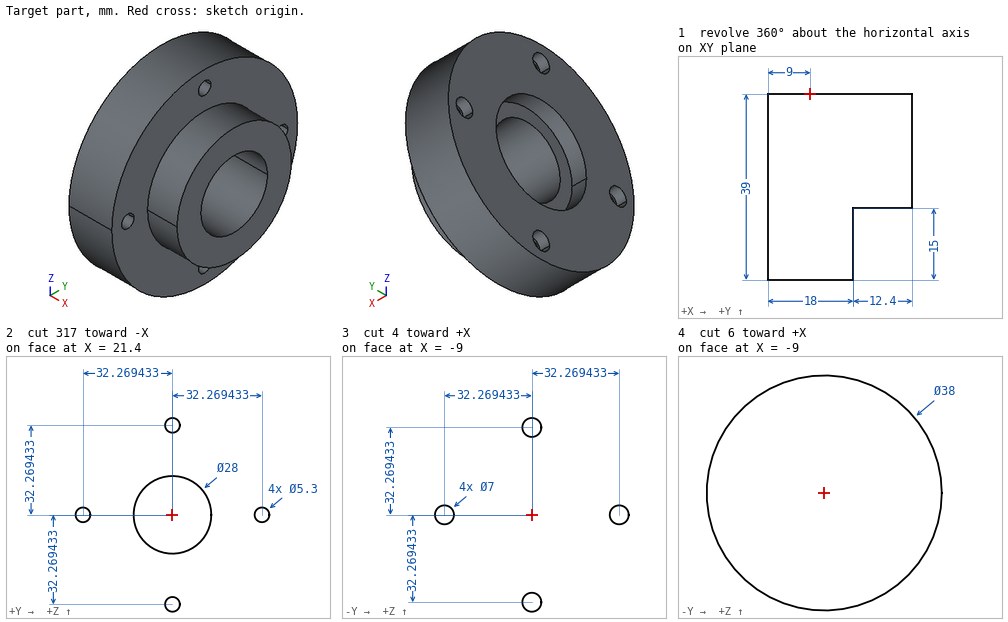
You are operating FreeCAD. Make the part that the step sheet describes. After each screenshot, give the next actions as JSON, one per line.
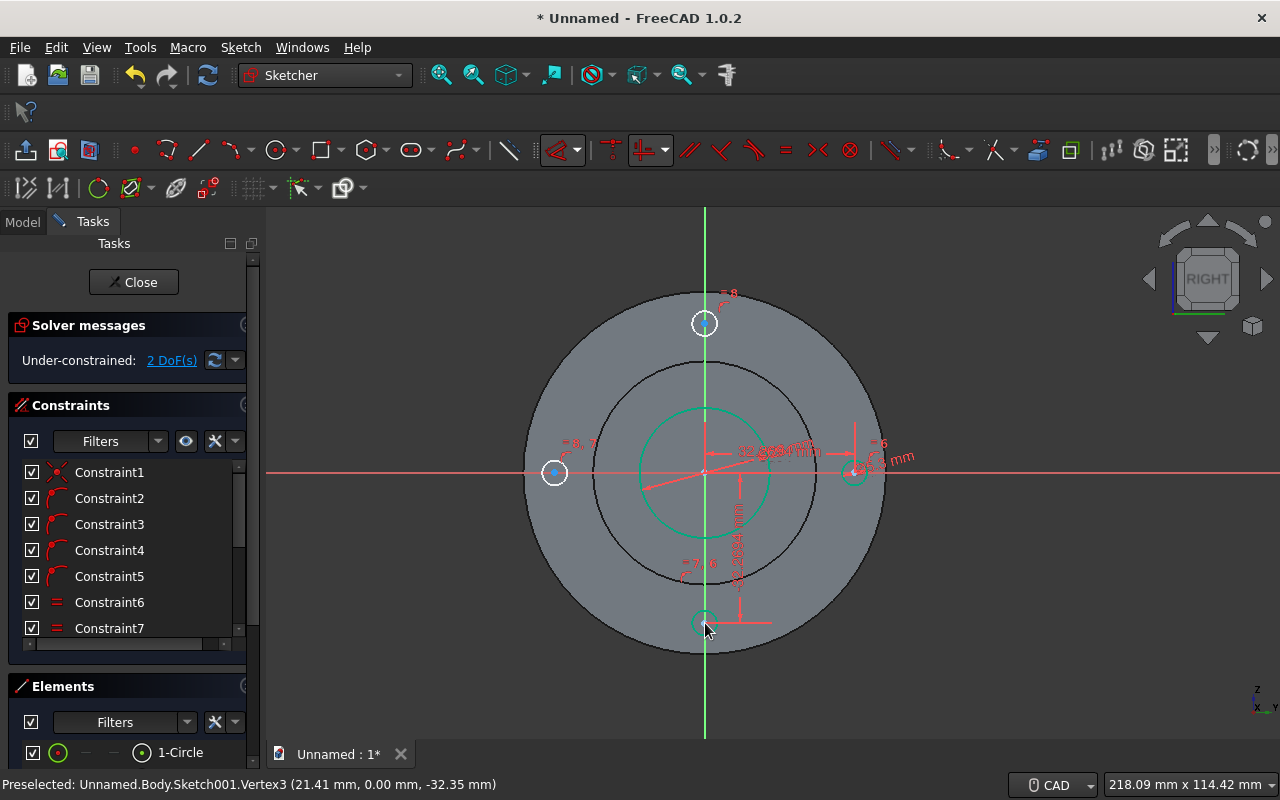
{"action": "left_click", "coordinate": [555, 473]}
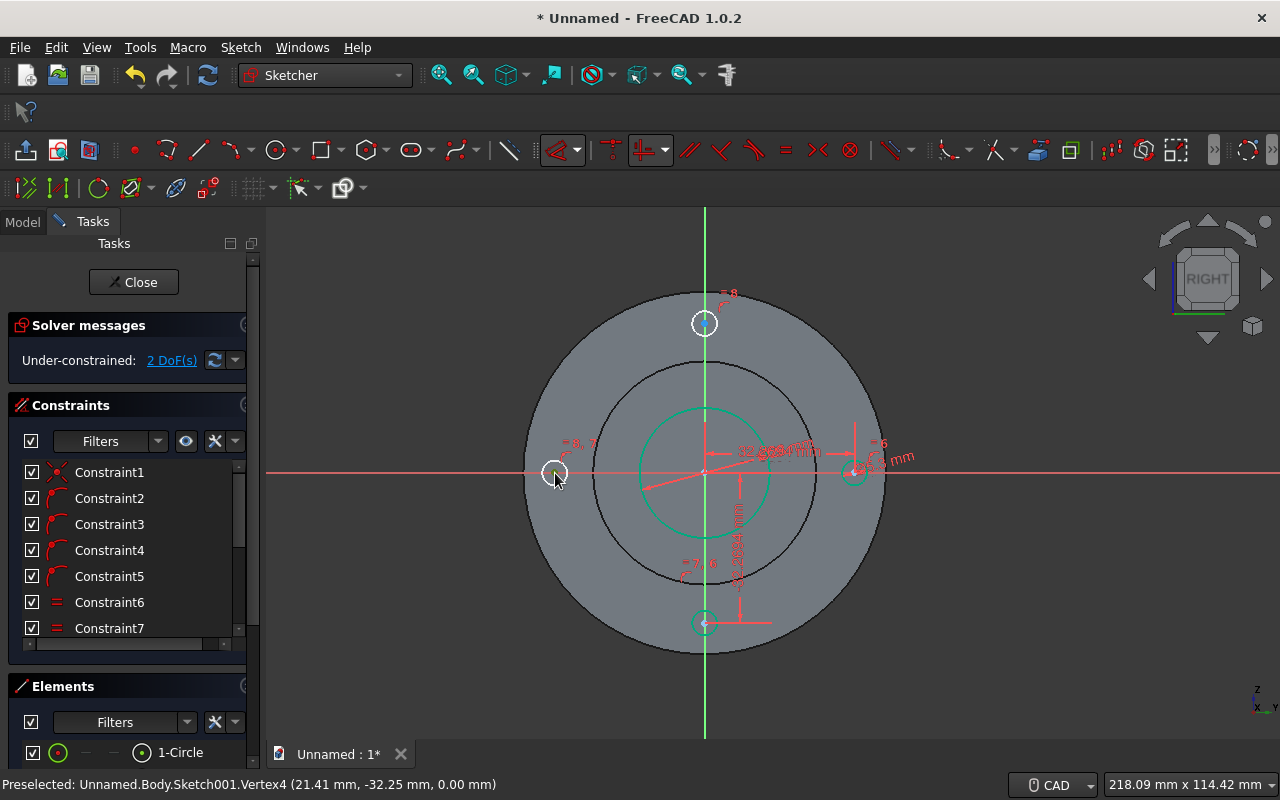
{"action": "left_click", "coordinate": [580, 150]}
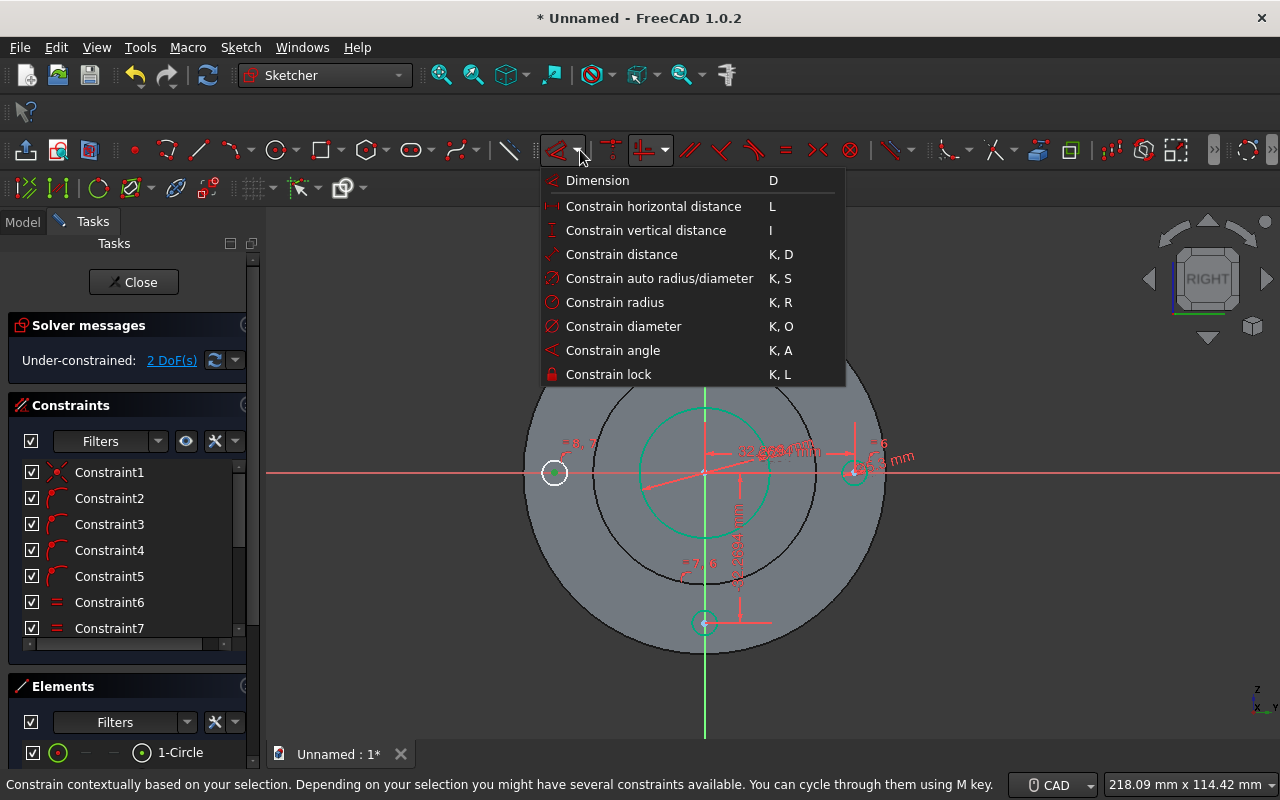
{"action": "left_click", "coordinate": [693, 206]}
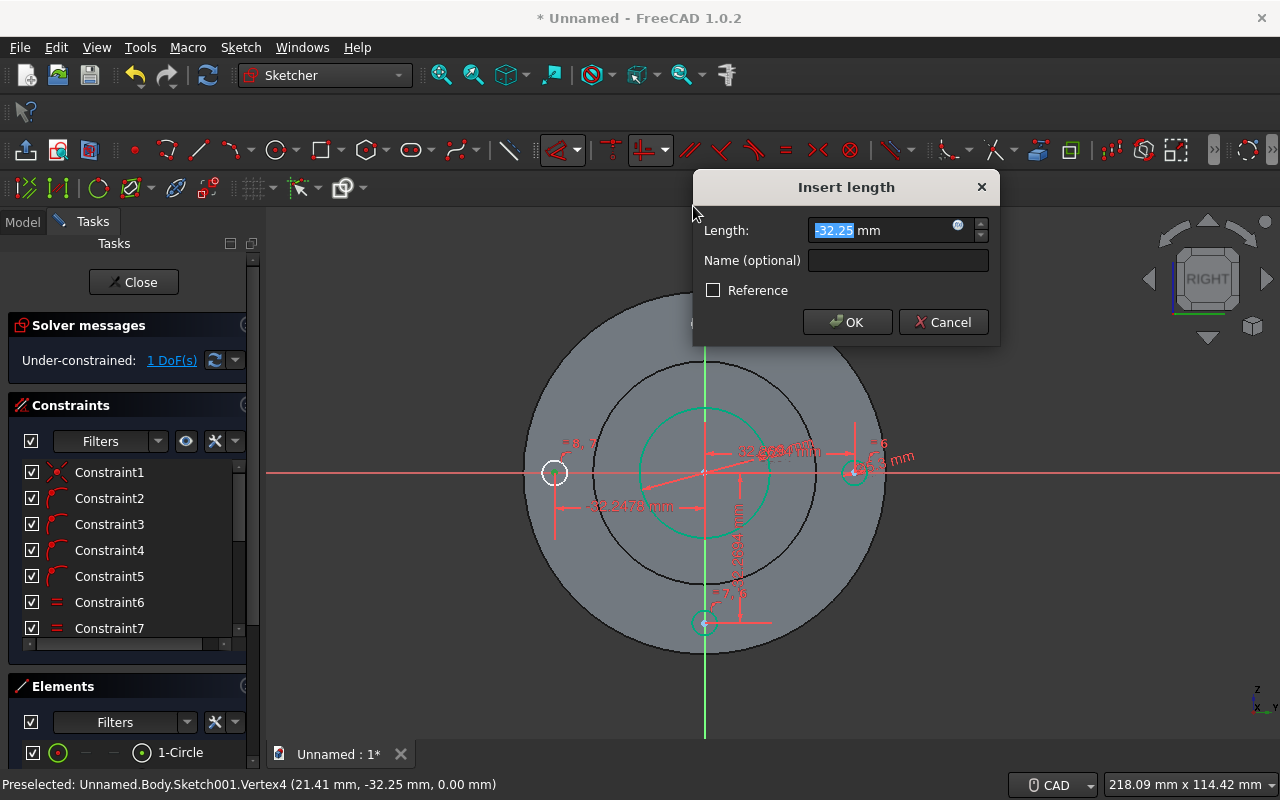
{"action": "type", "text": "-32.269433"}
{"action": "key", "text": "Return"}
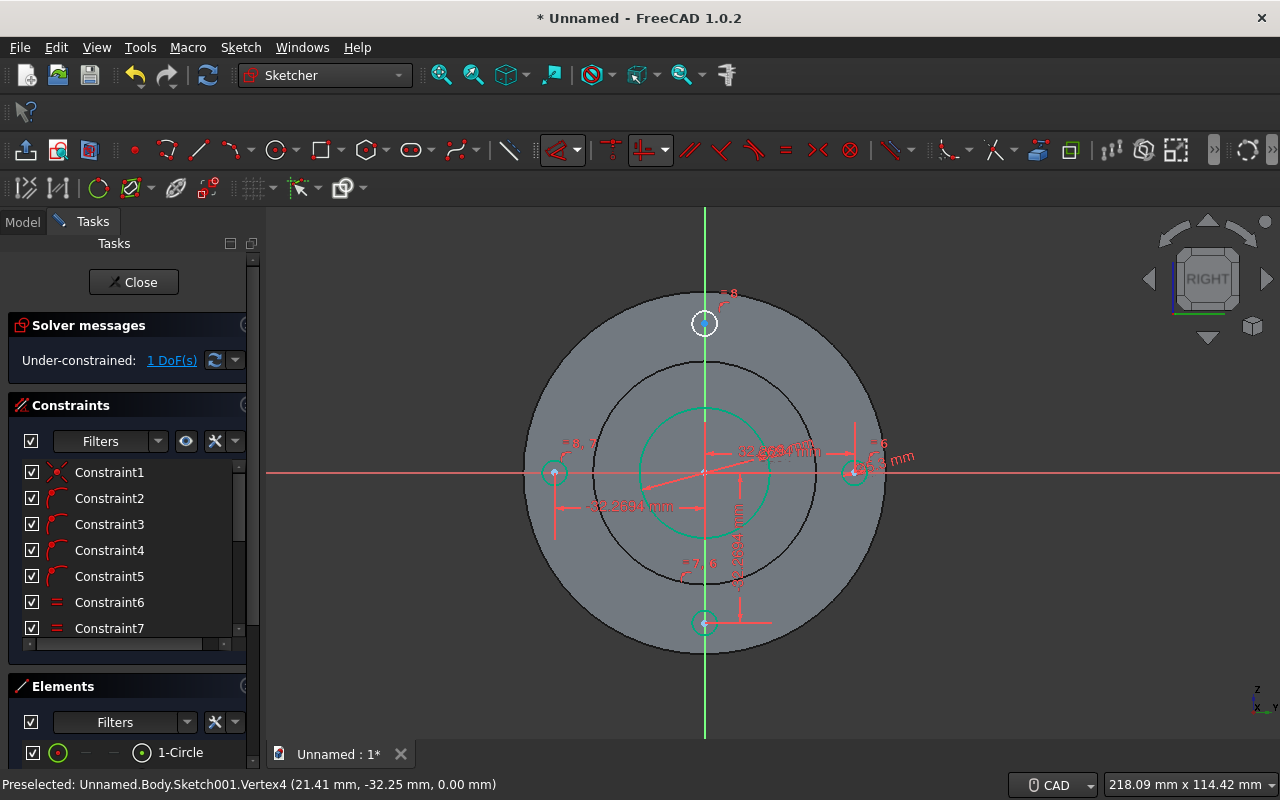
{"action": "left_click", "coordinate": [705, 324]}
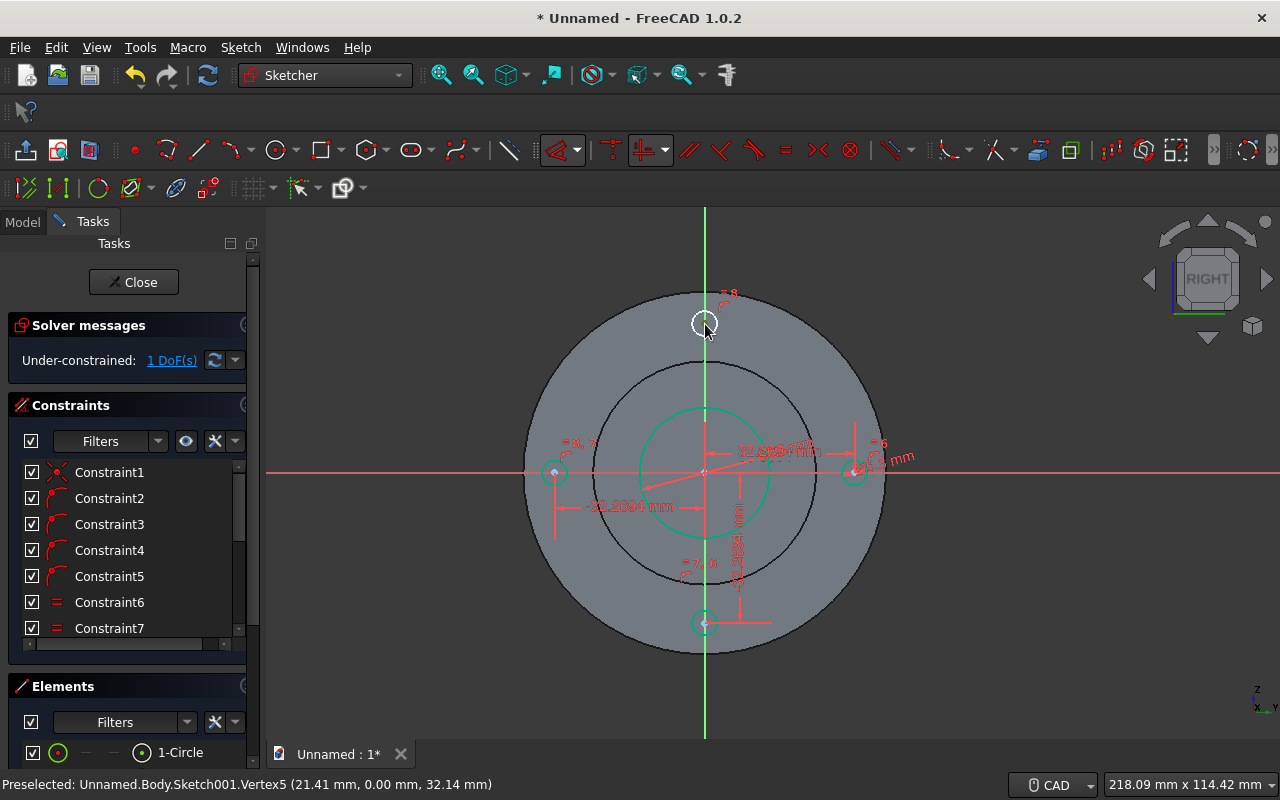
{"action": "left_click", "coordinate": [580, 150]}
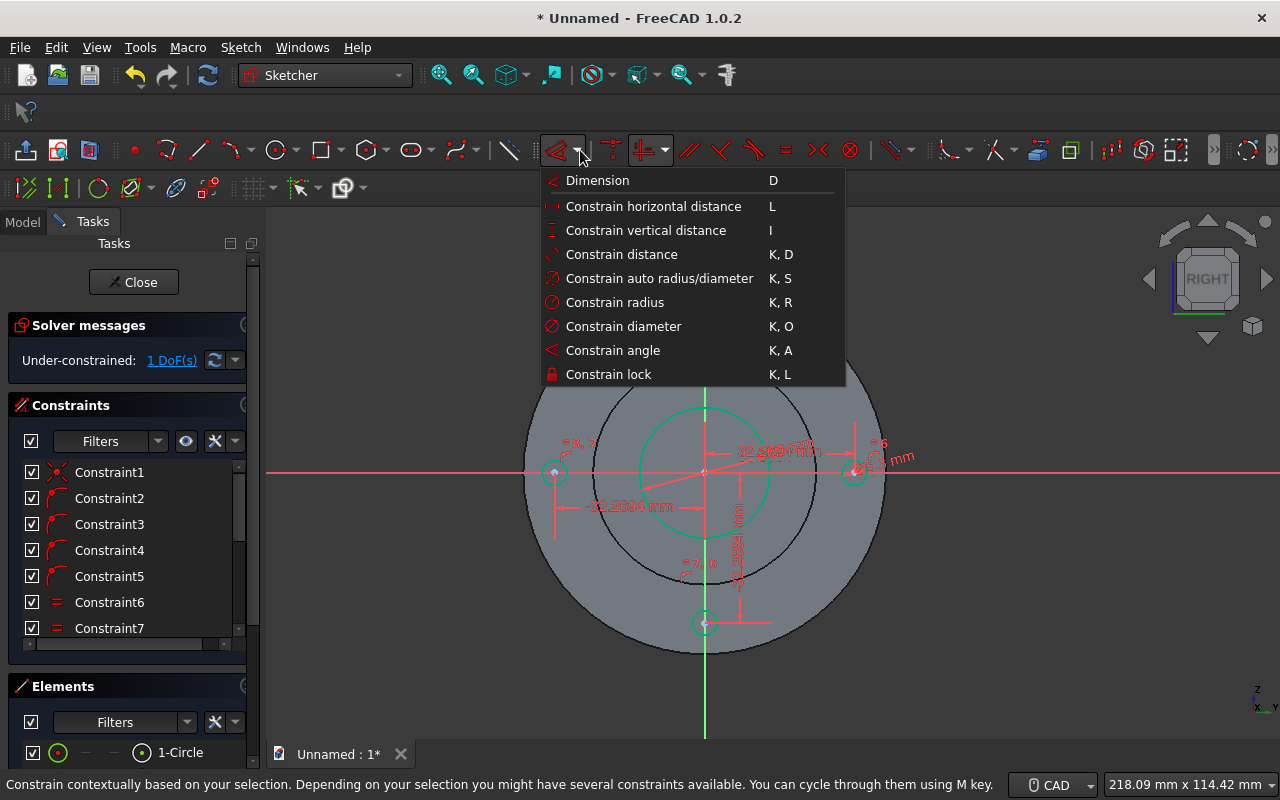
{"action": "left_click", "coordinate": [693, 230]}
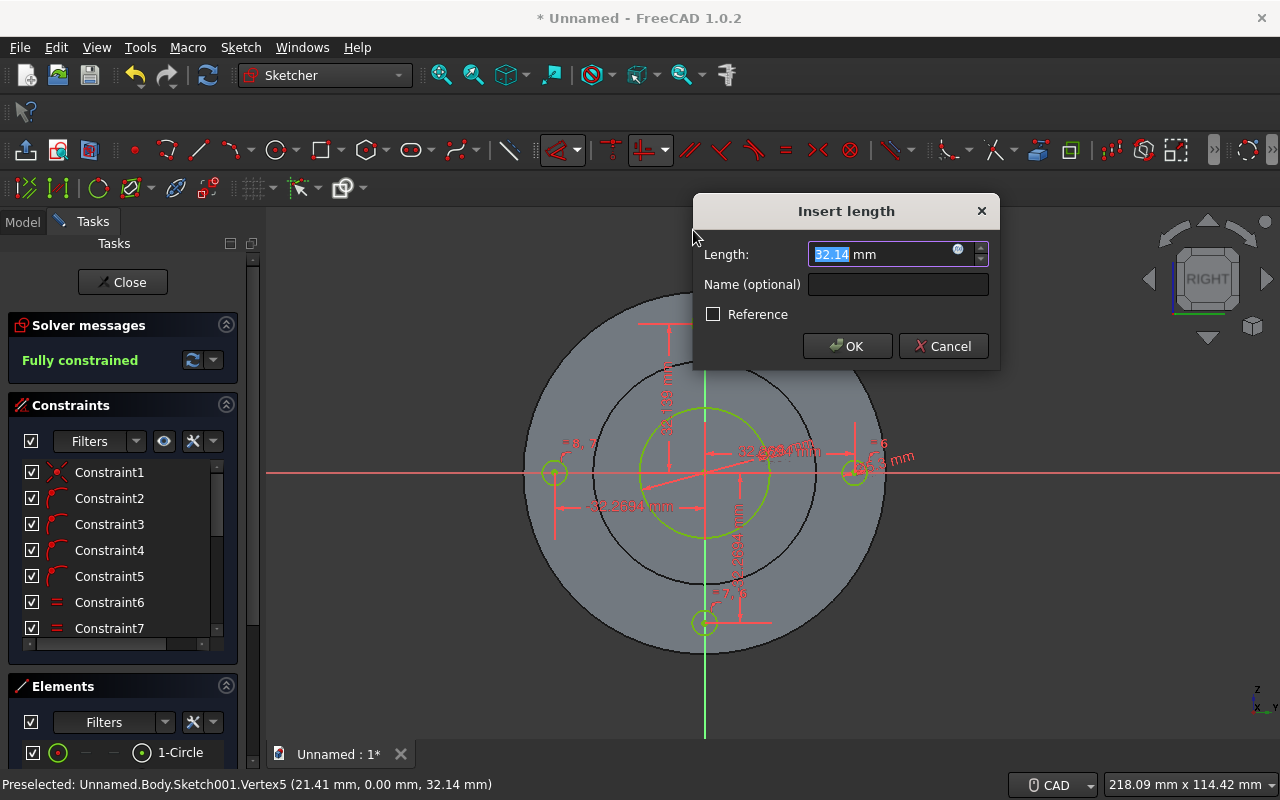
{"action": "type", "text": "32.269433"}
{"action": "key", "text": "Return"}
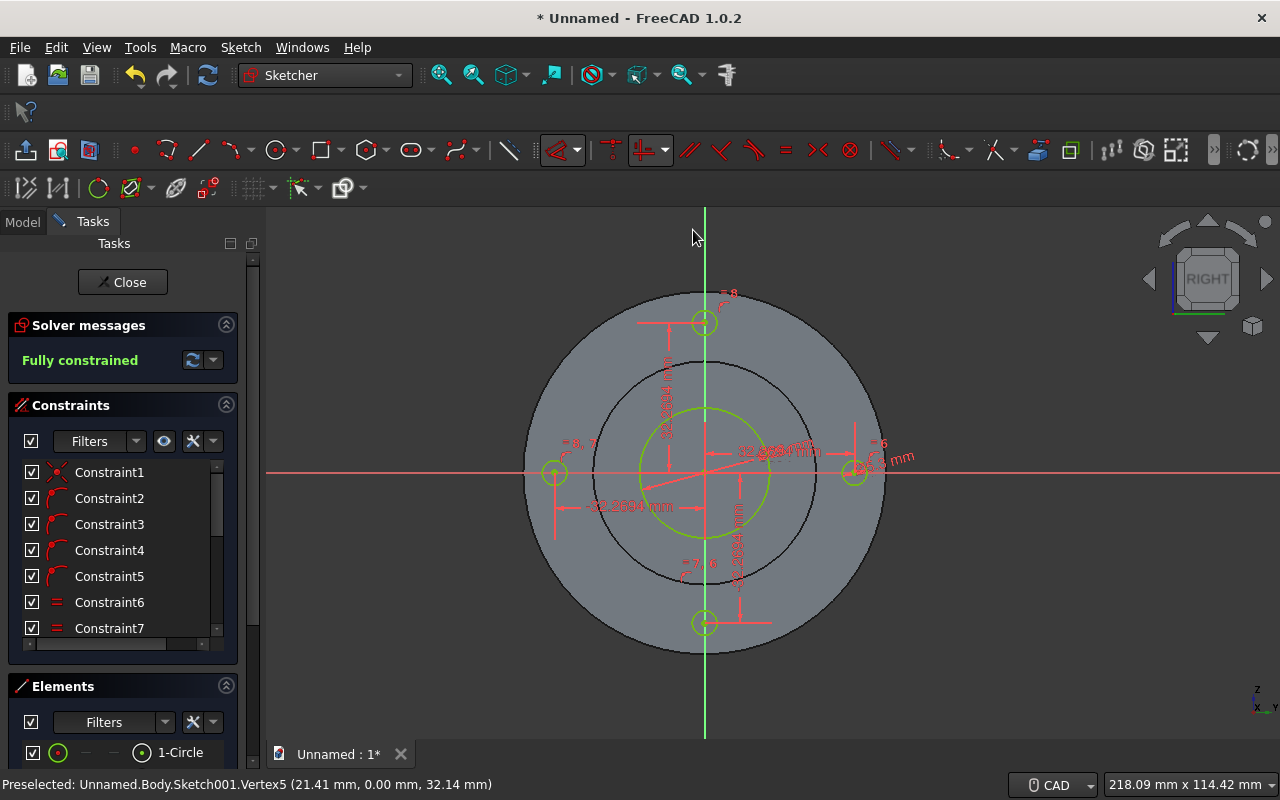
{"action": "left_click", "coordinate": [123, 282]}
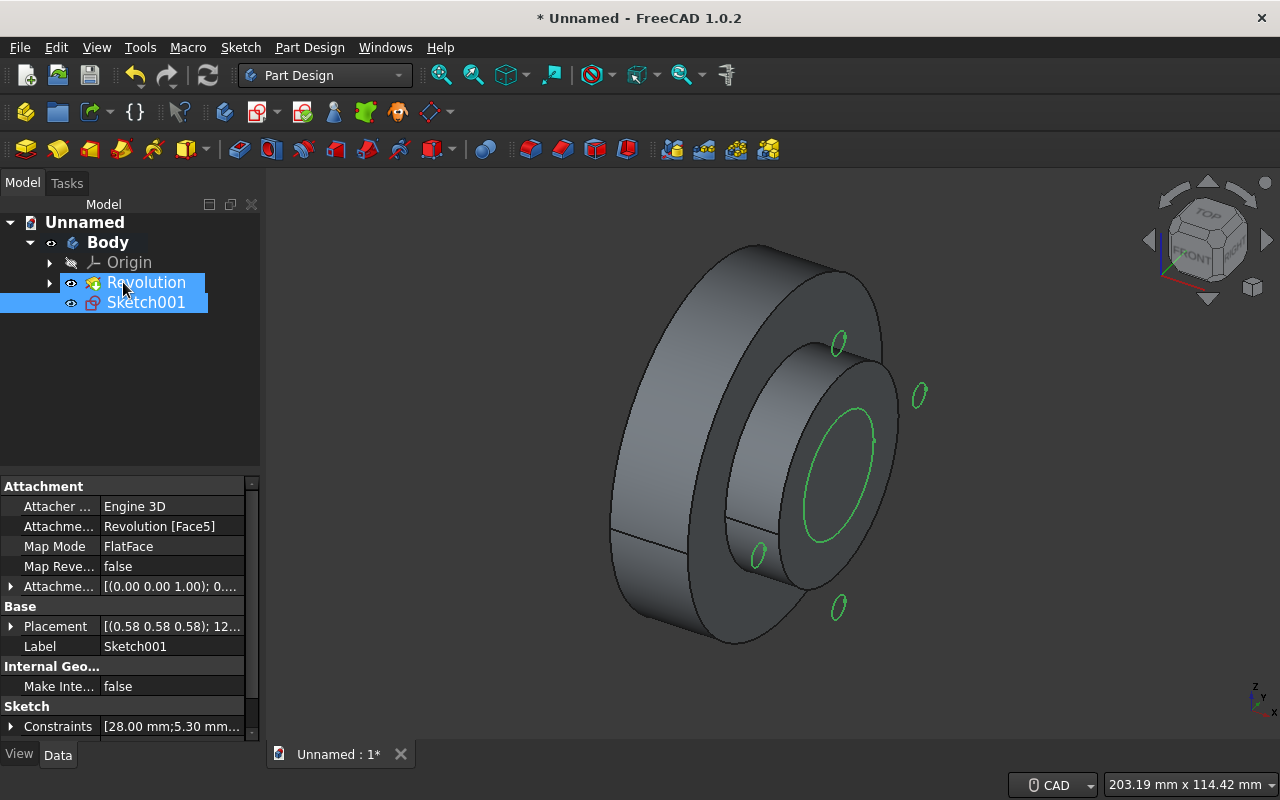
{"action": "left_click", "coordinate": [240, 150]}